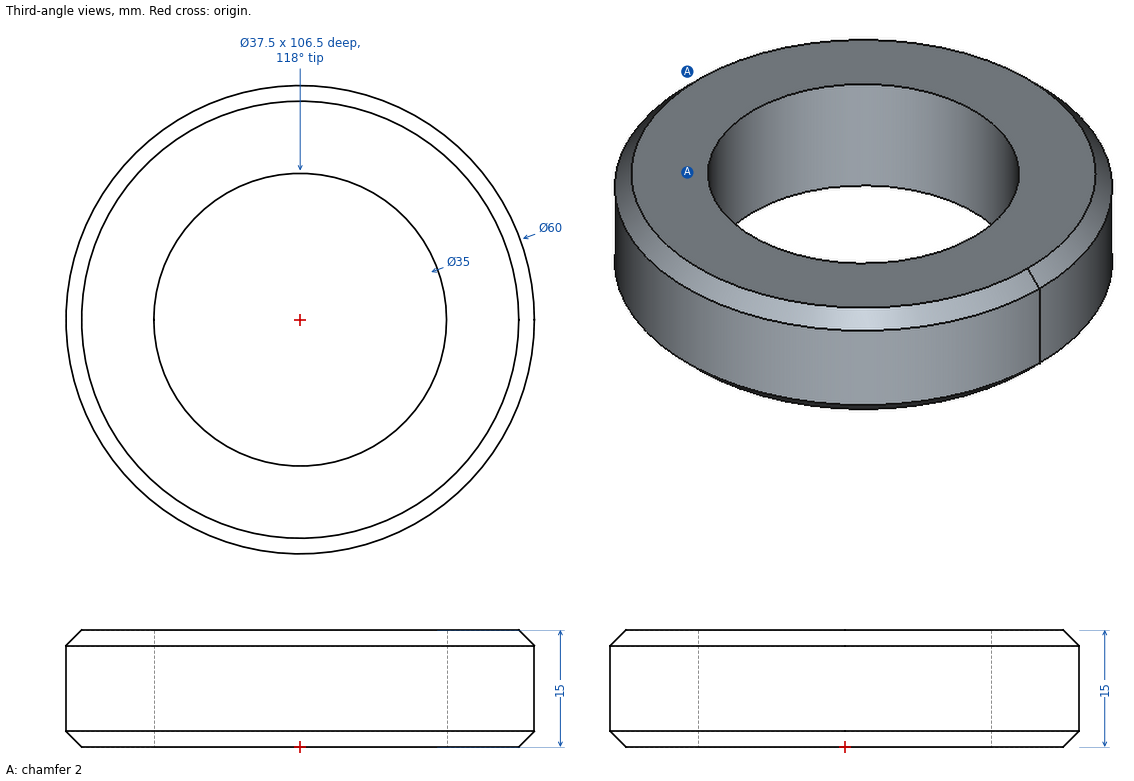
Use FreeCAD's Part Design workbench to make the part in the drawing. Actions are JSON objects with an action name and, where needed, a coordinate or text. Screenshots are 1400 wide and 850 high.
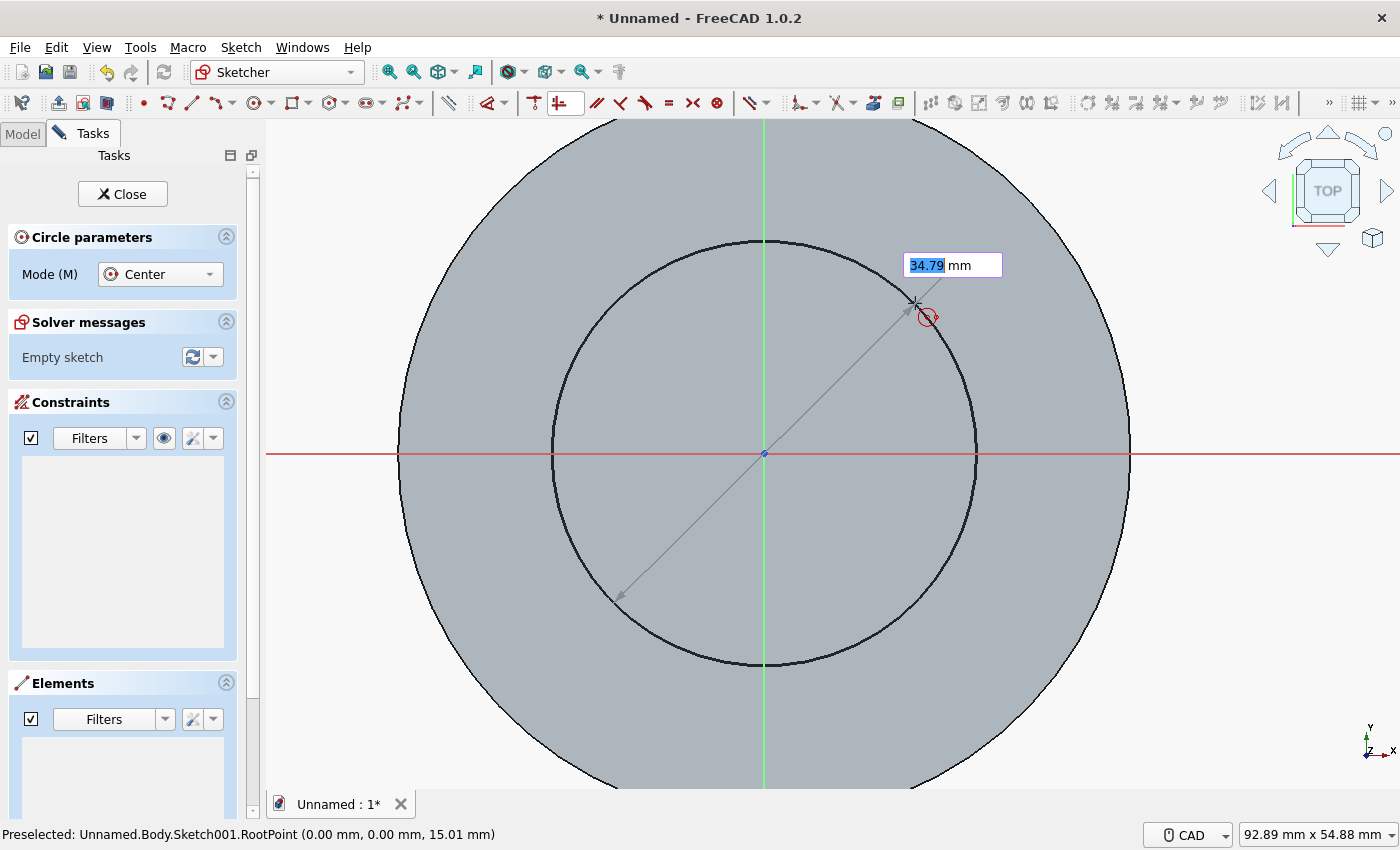
{"action": "type", "text": "35"}
{"action": "key", "text": "Return"}
{"action": "key", "text": "Escape"}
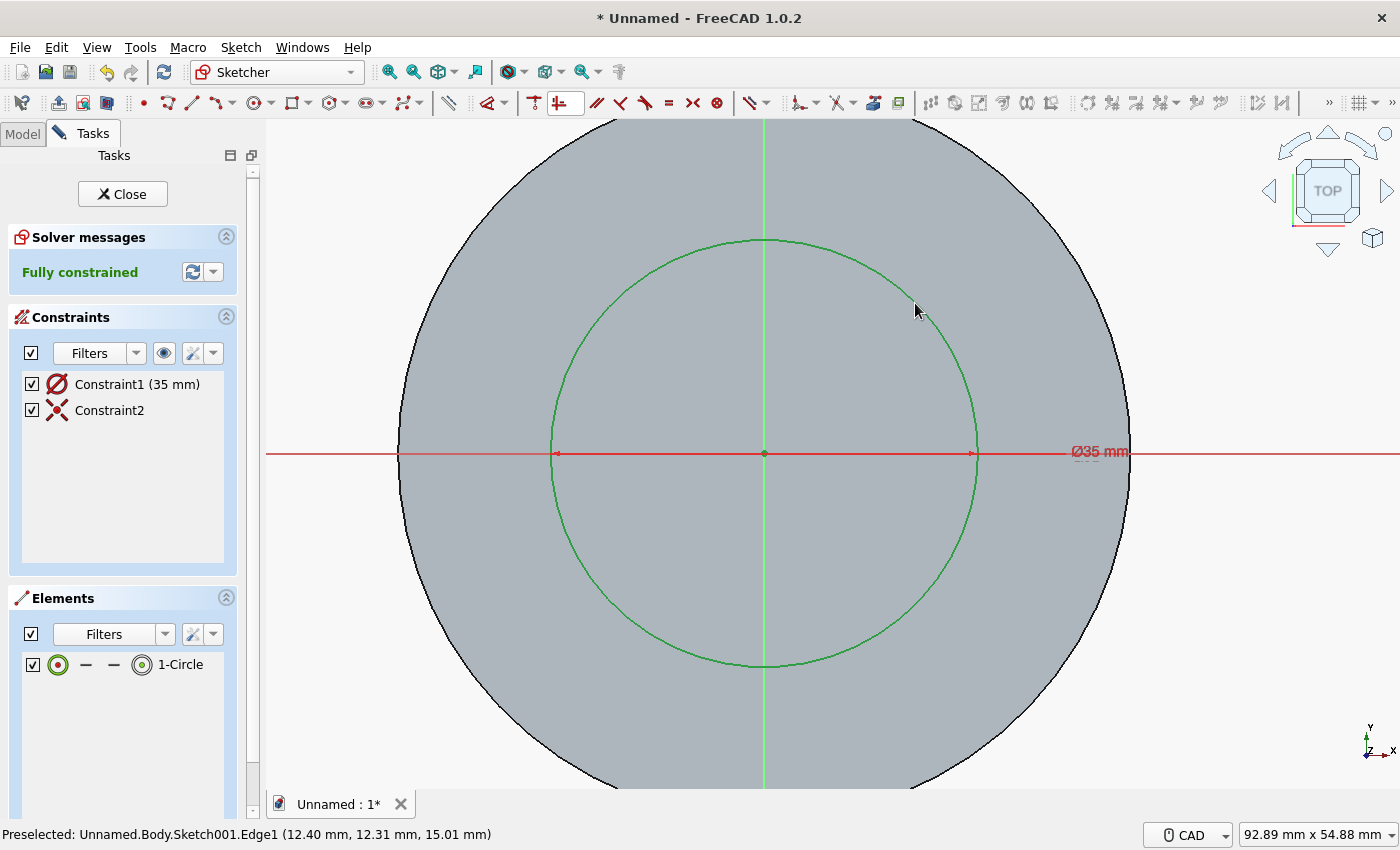
{"action": "left_click", "coordinate": [123, 194]}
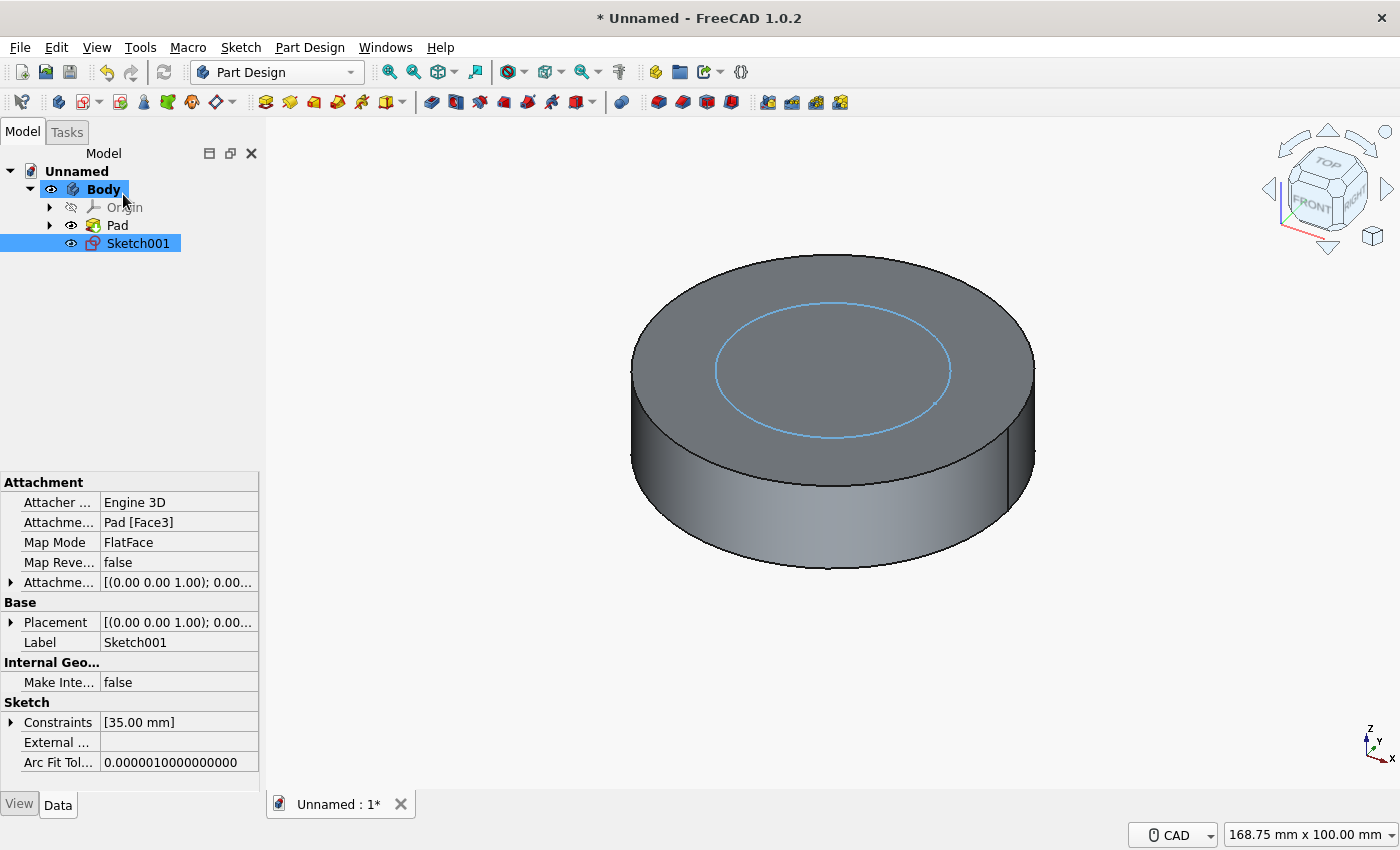
{"action": "left_click", "coordinate": [432, 102]}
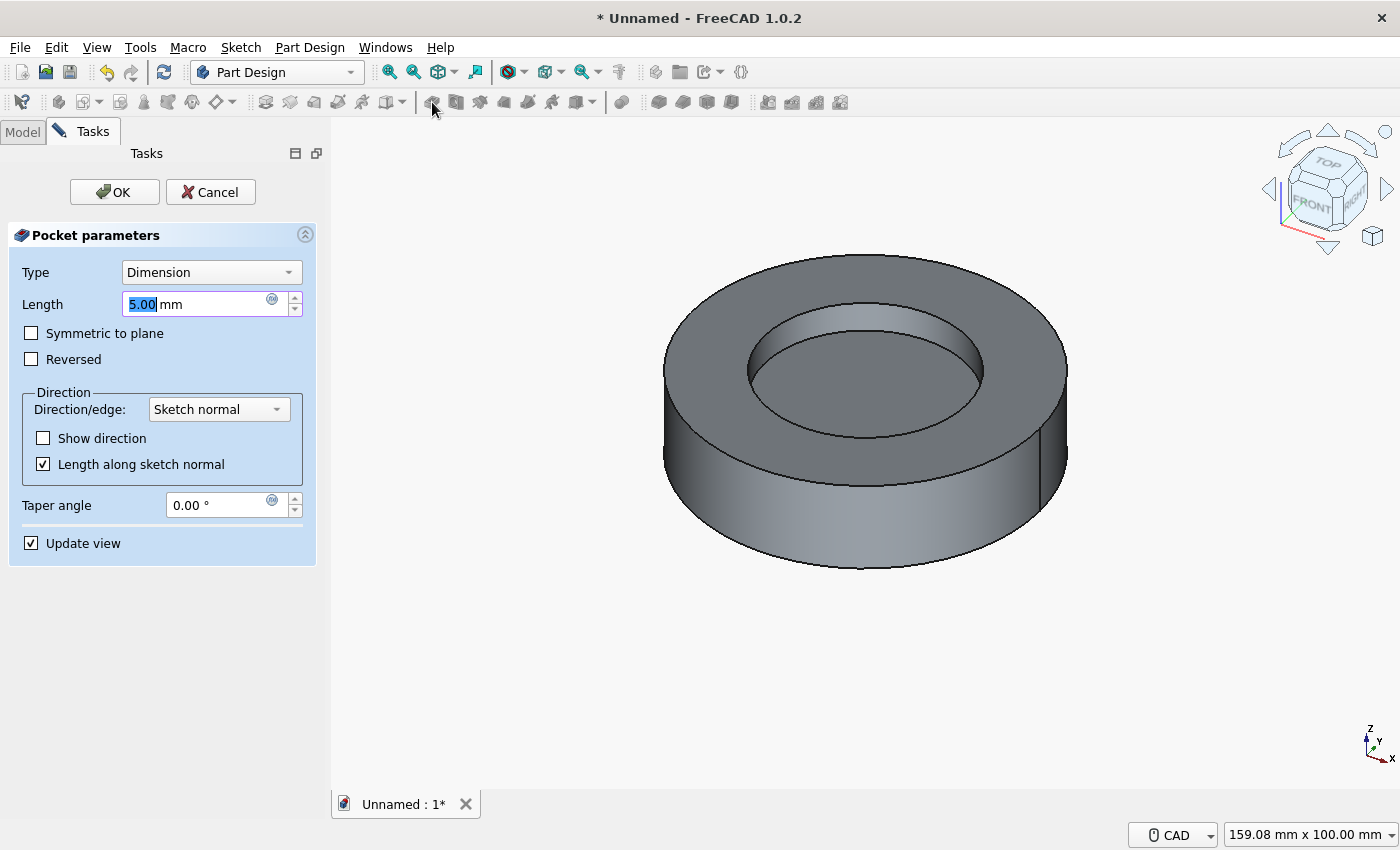
{"action": "type", "text": "15"}
{"action": "key", "text": "Tab"}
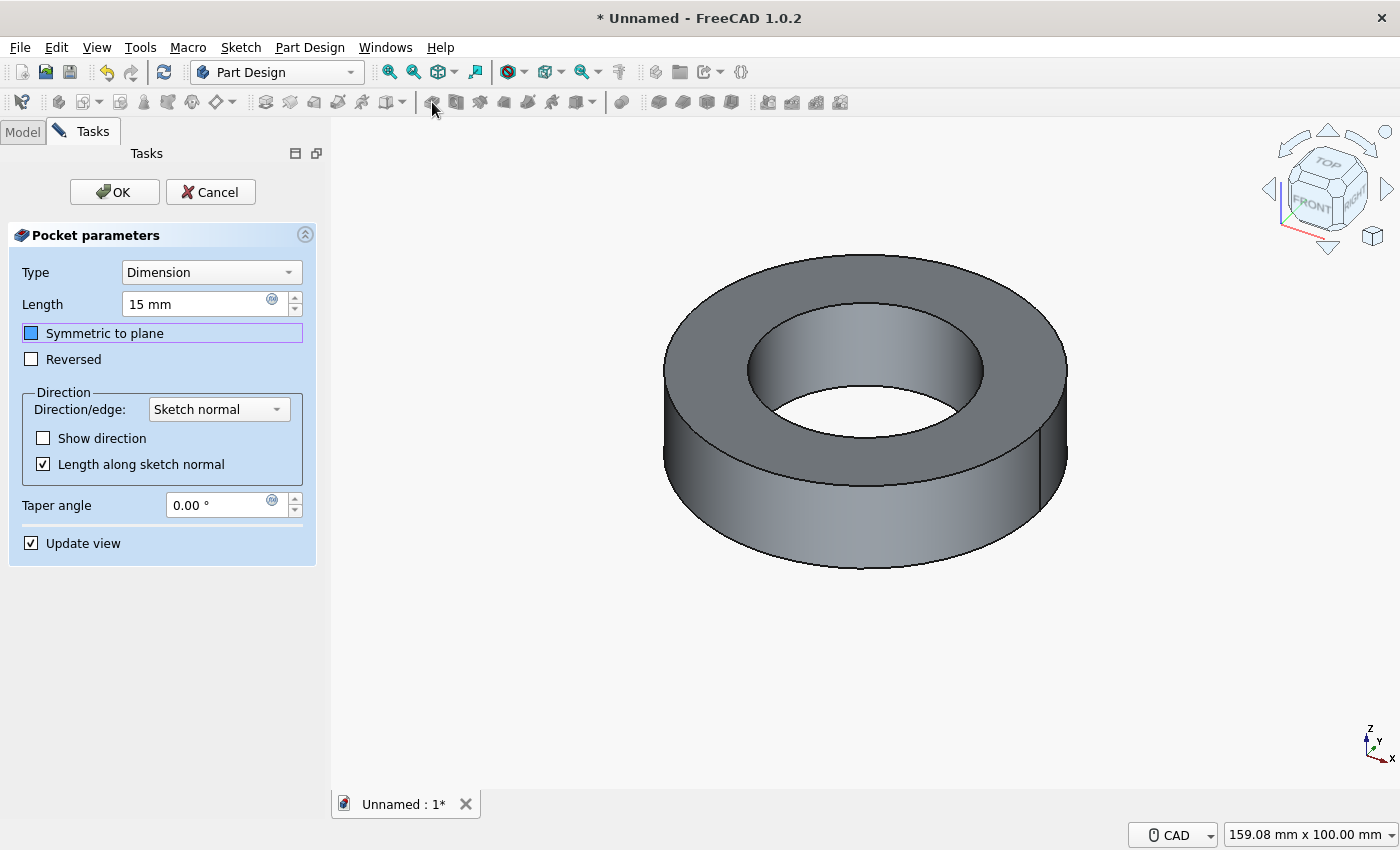
{"action": "left_click", "coordinate": [115, 192]}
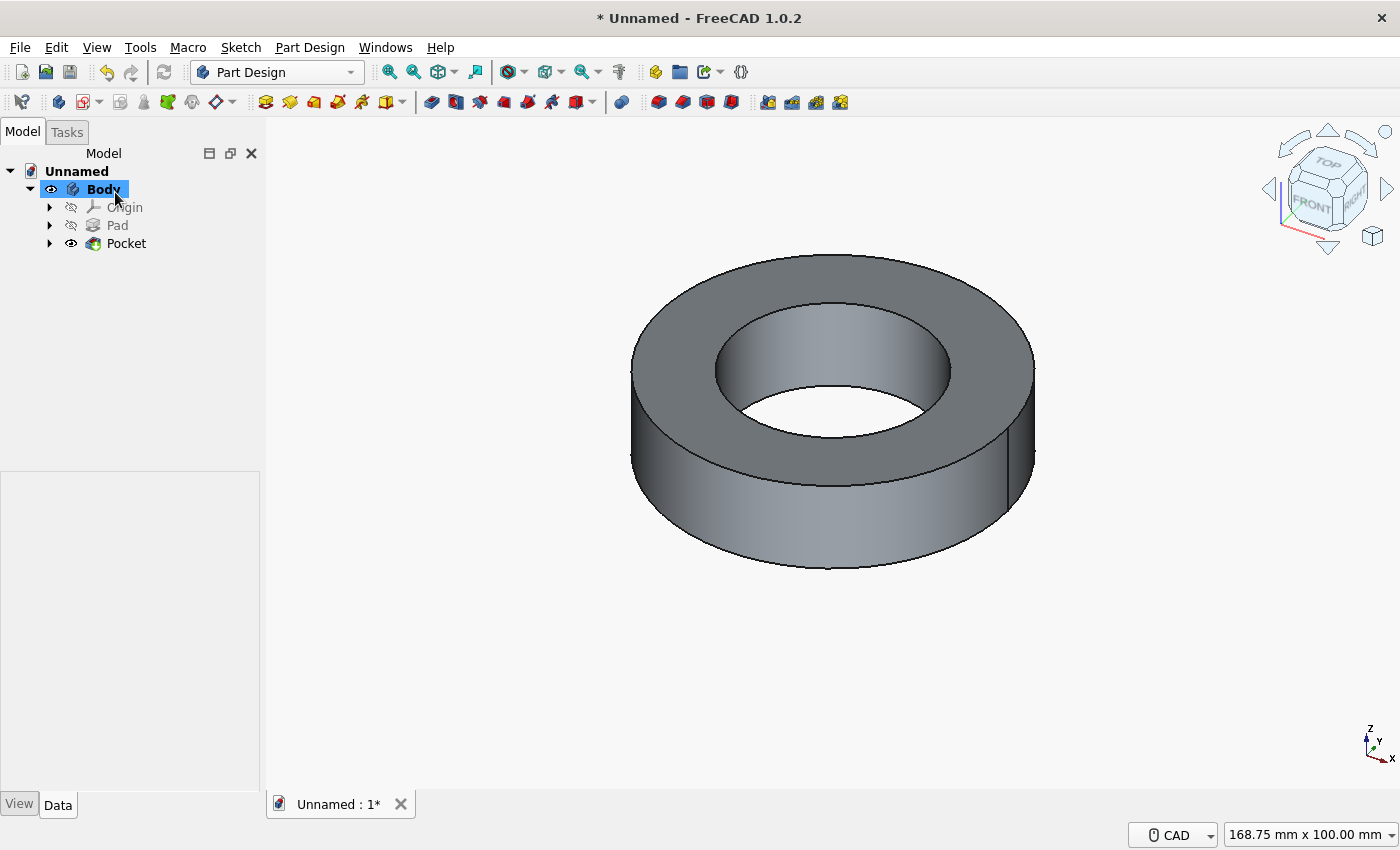
{"action": "left_click", "coordinate": [633, 382]}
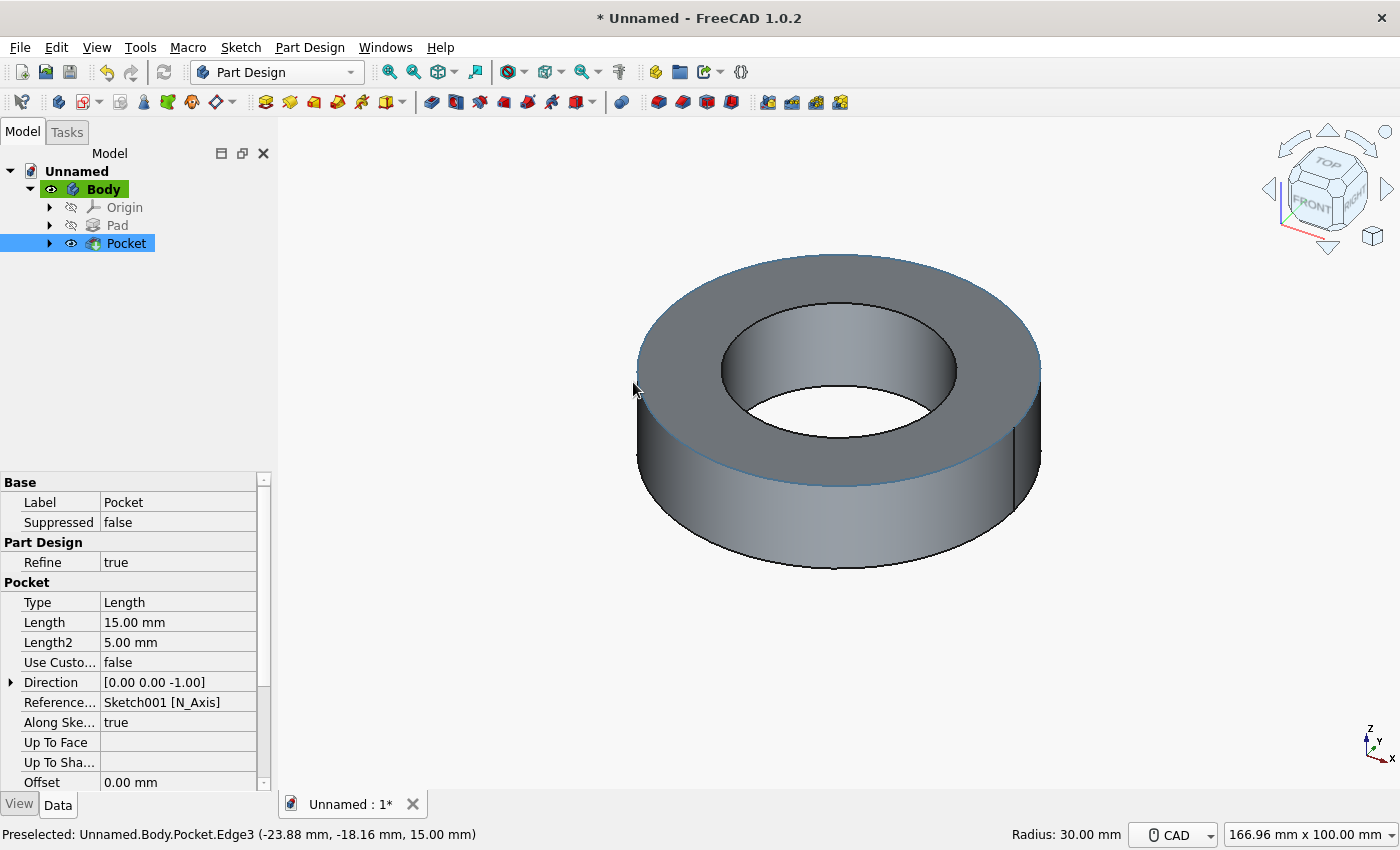
{"action": "key", "text": "0"}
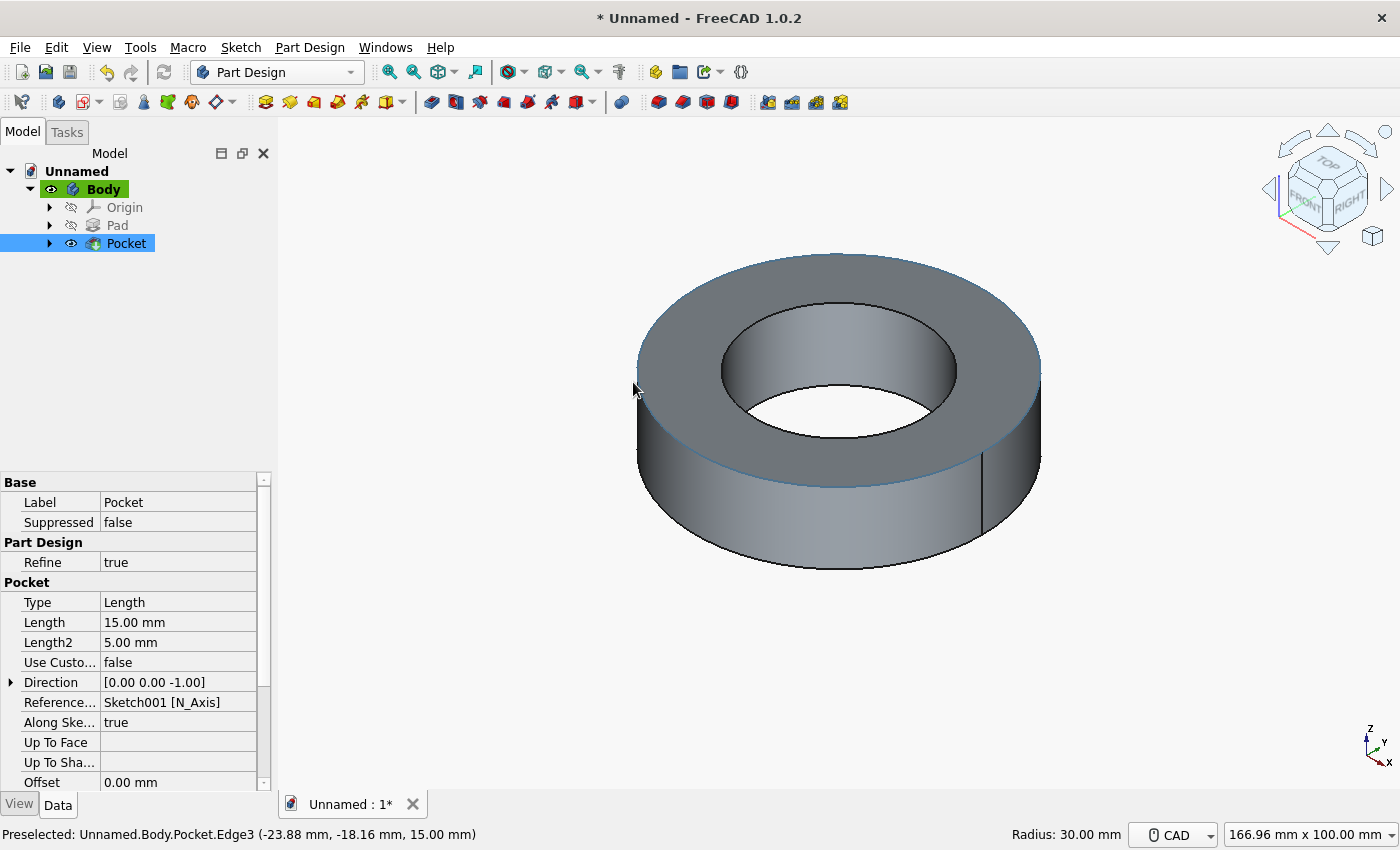
{"action": "key", "text": "2"}